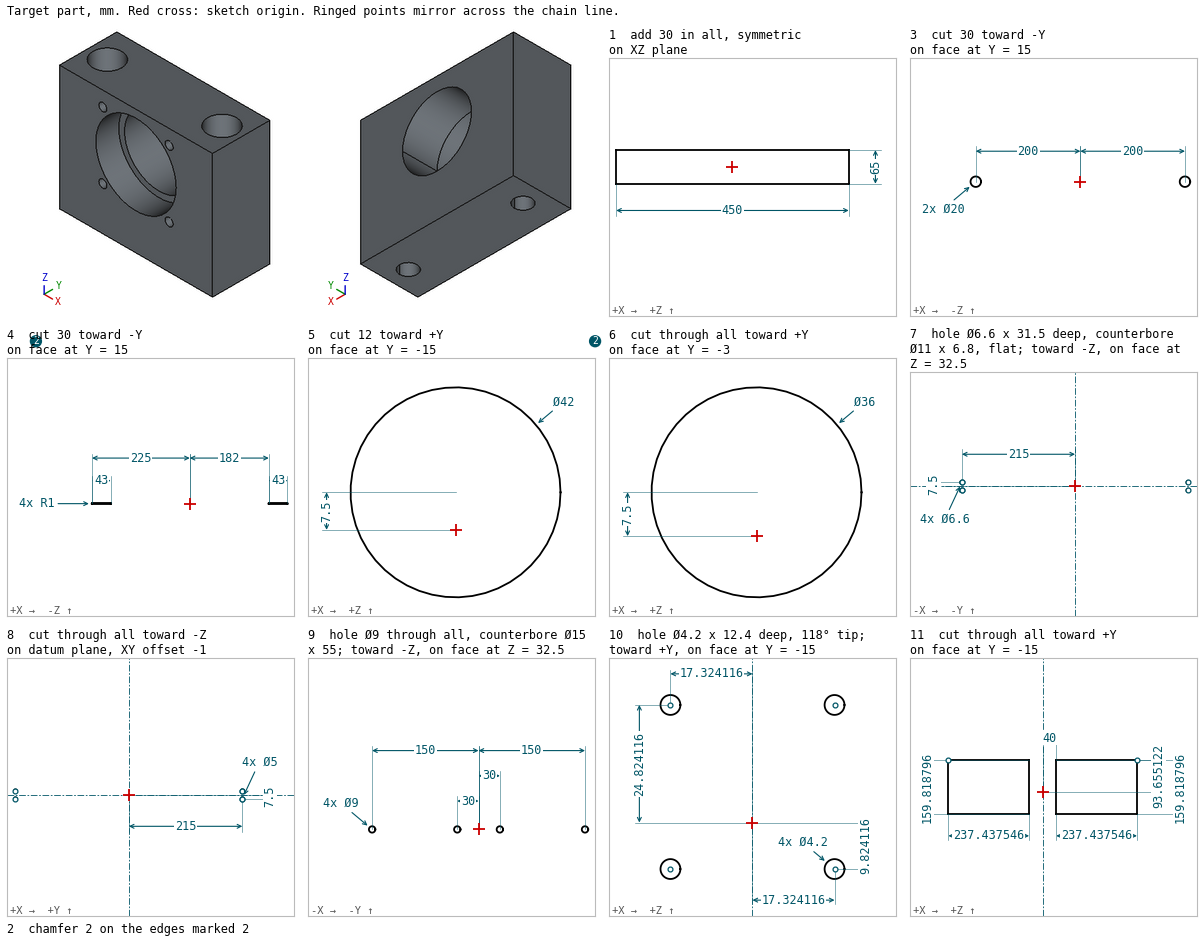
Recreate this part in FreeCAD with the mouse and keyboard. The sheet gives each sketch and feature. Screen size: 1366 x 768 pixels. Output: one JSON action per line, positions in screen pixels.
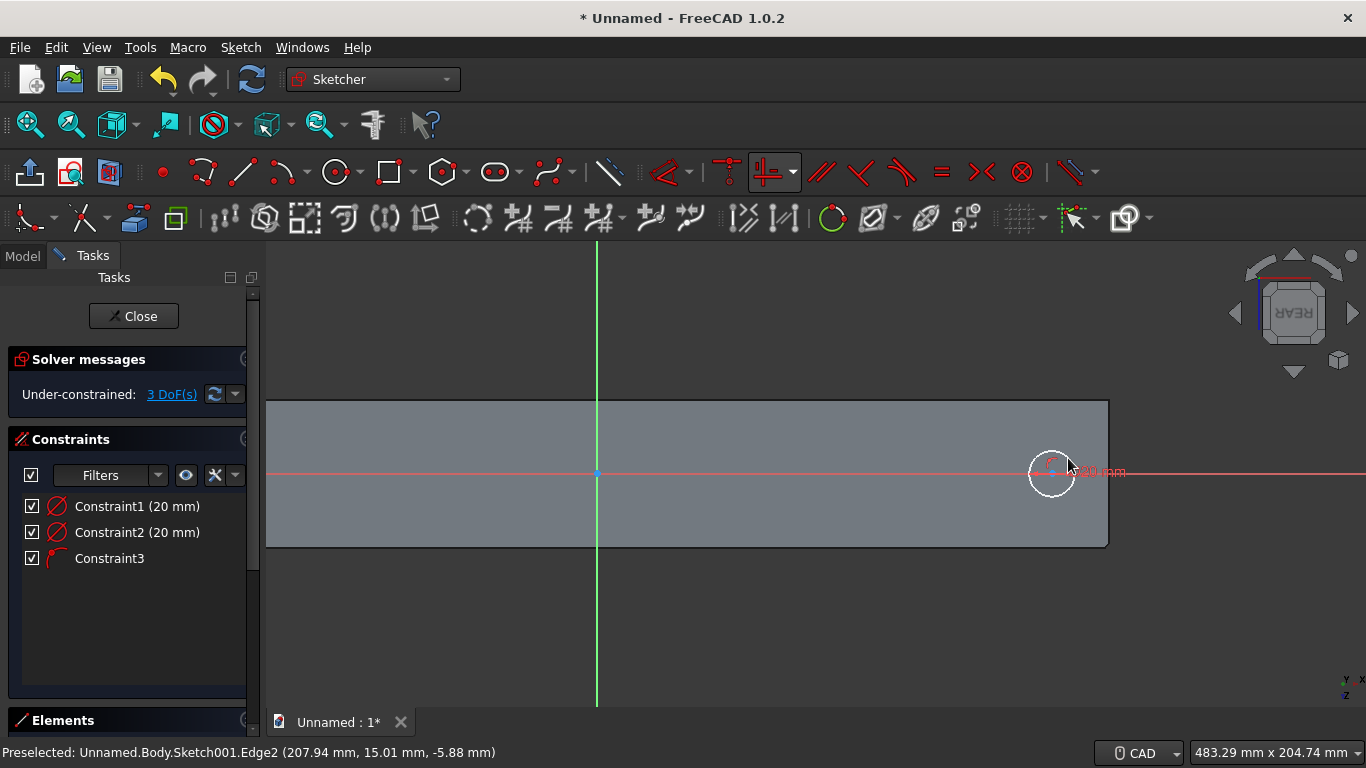
{"action": "scroll", "coordinate": [1053, 474], "scroll_direction": "down", "scroll_amount": 2}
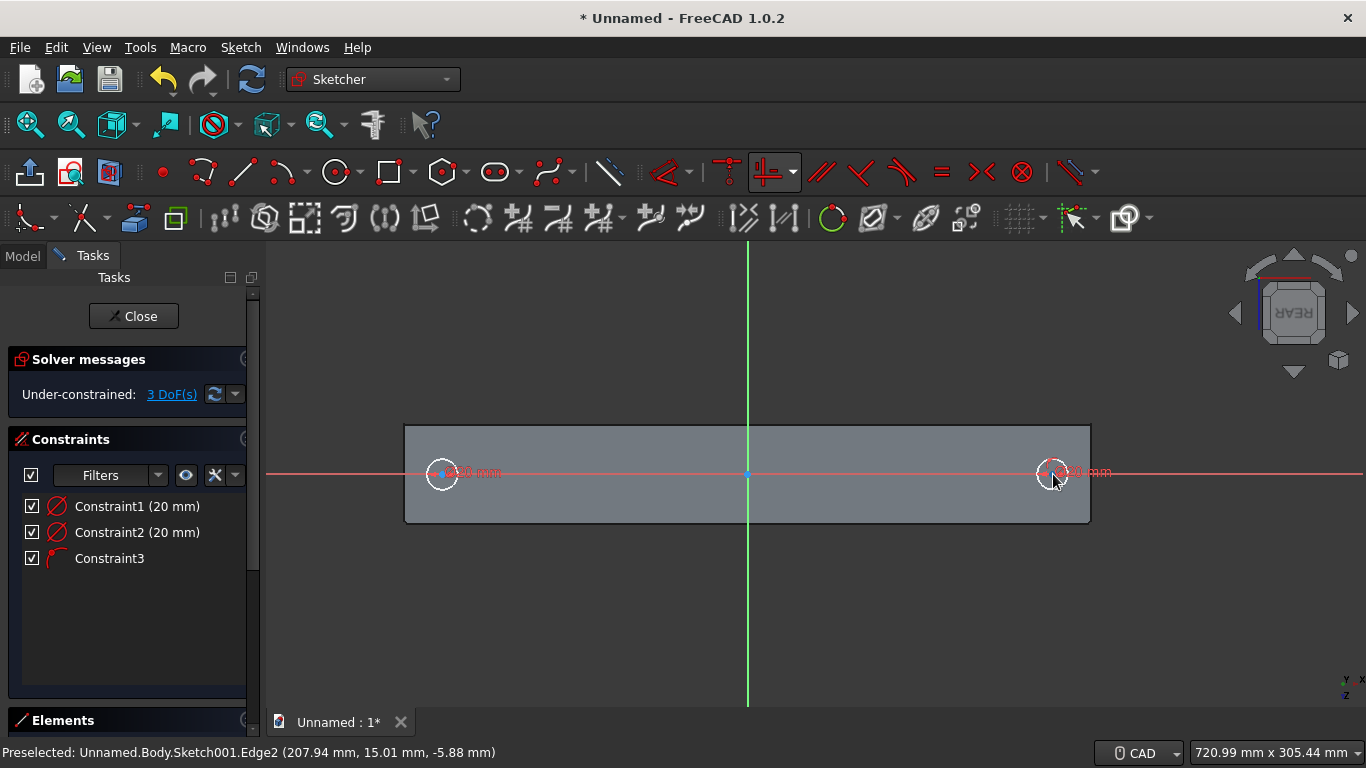
{"action": "left_click", "coordinate": [442, 474]}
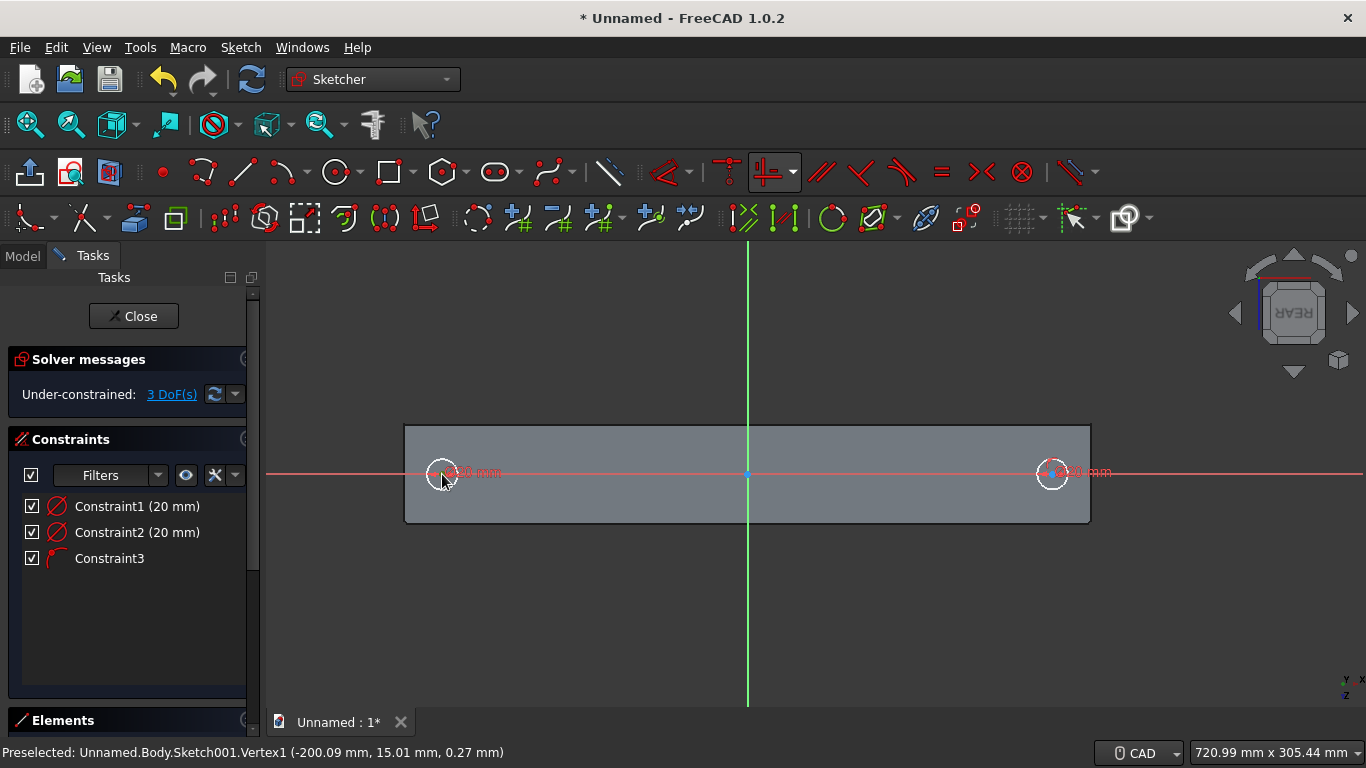
{"action": "left_click", "coordinate": [359, 474]}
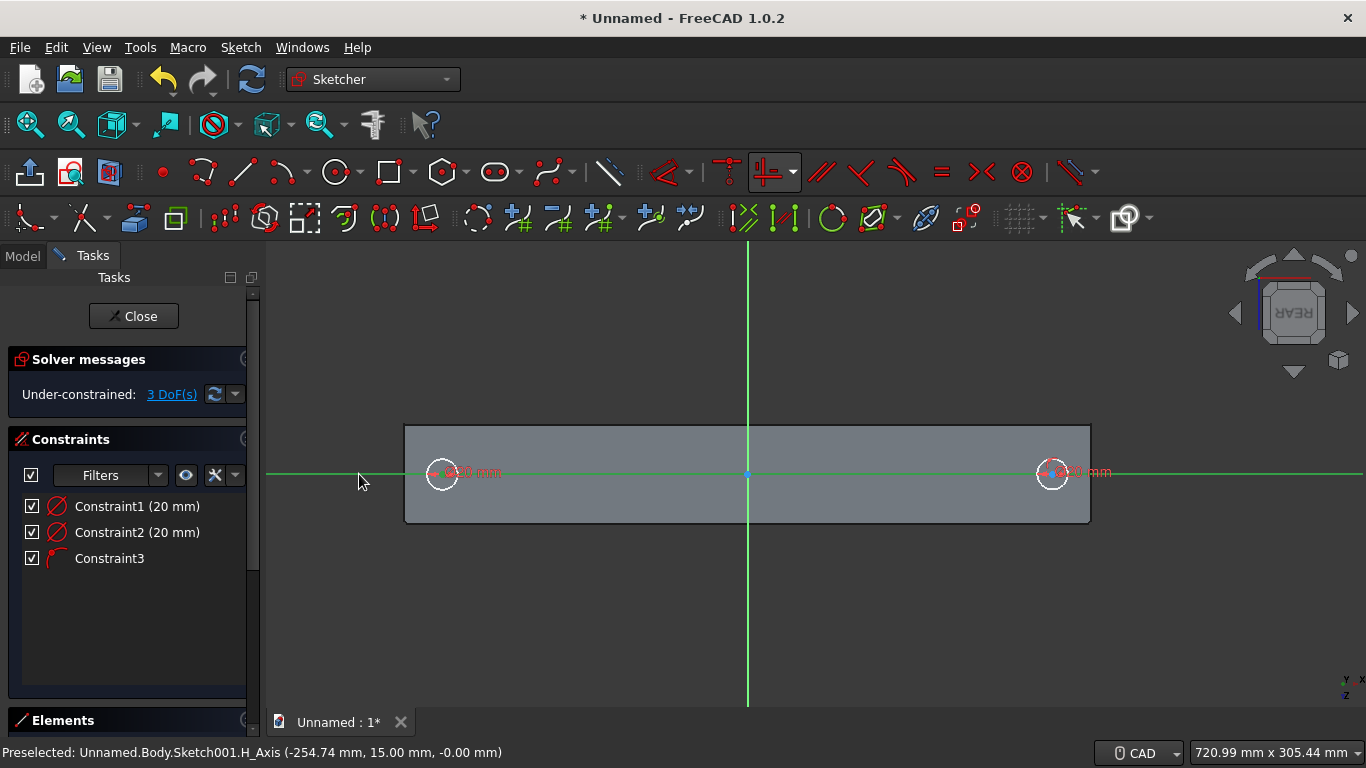
{"action": "key", "text": "c"}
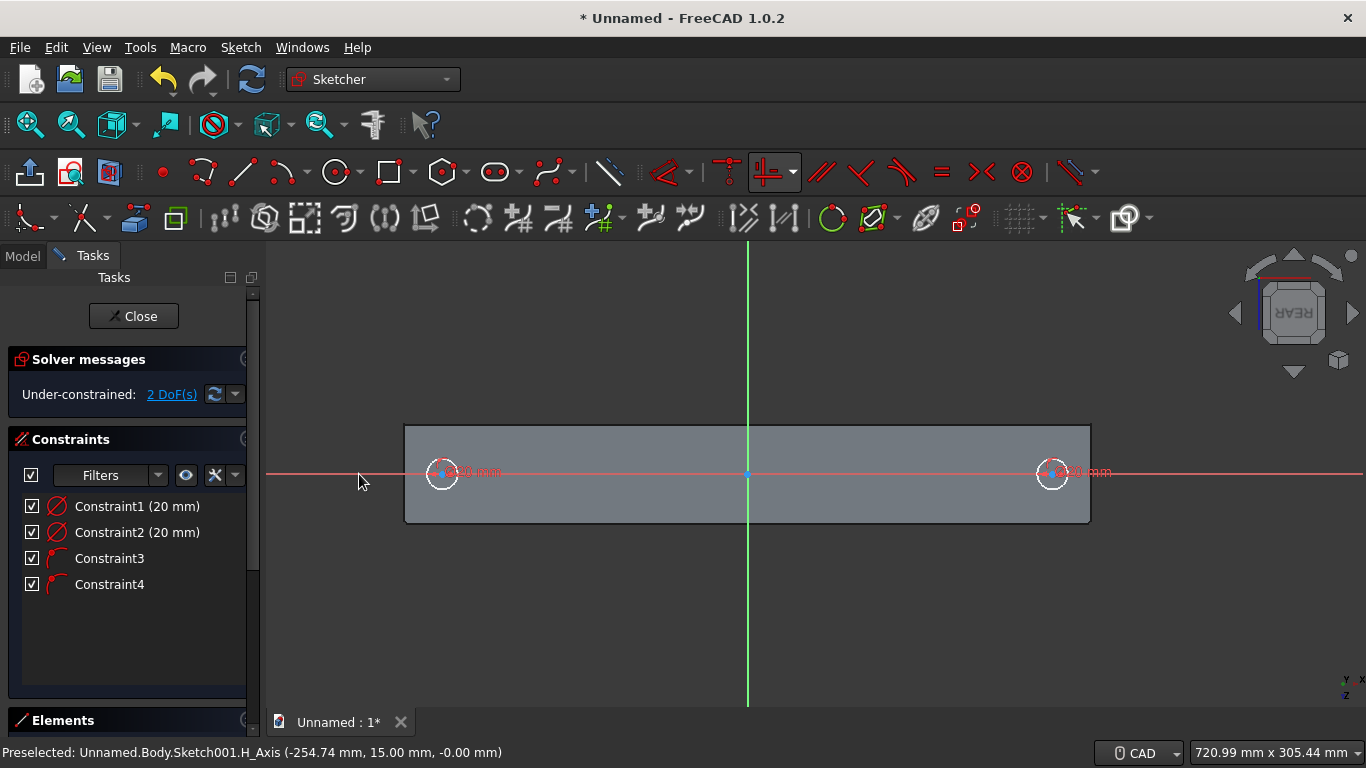
{"action": "key", "text": "d"}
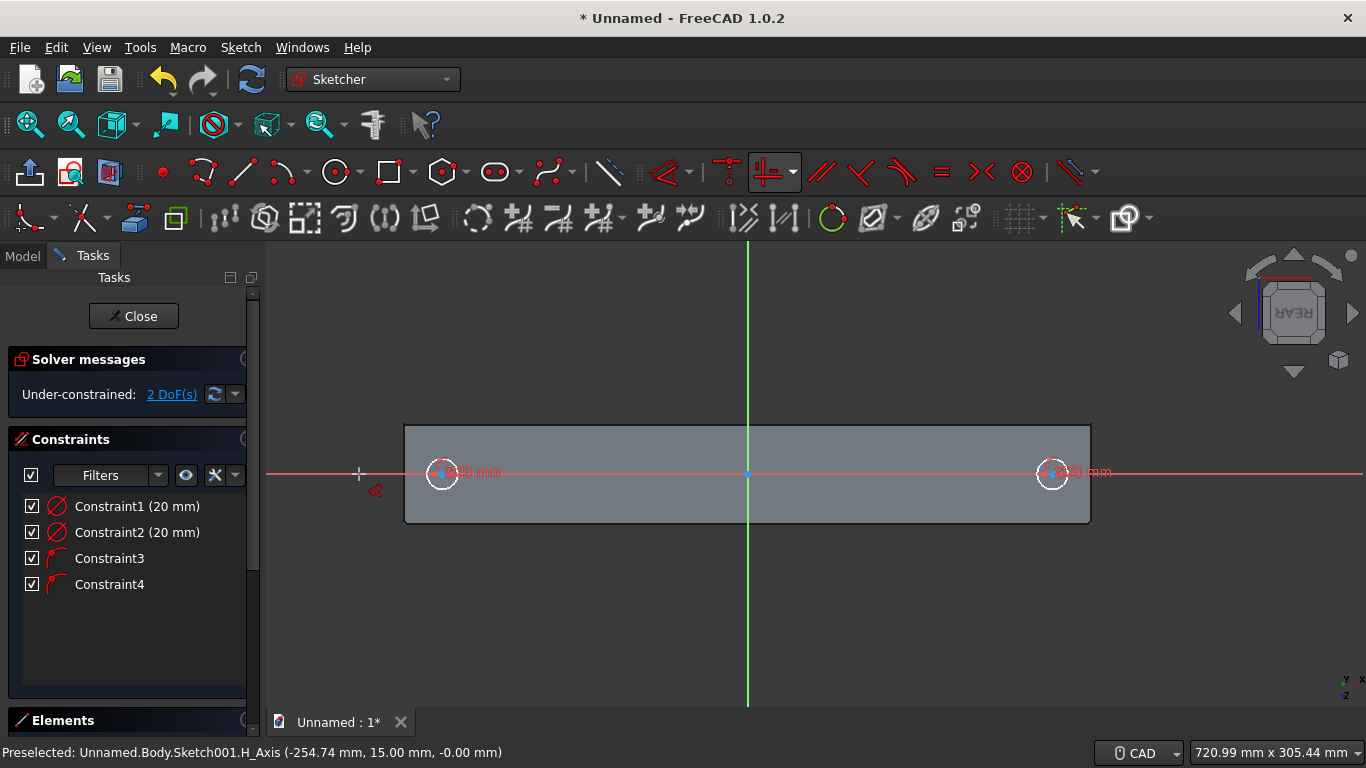
{"action": "left_click", "coordinate": [442, 474]}
{"action": "left_click", "coordinate": [595, 508]}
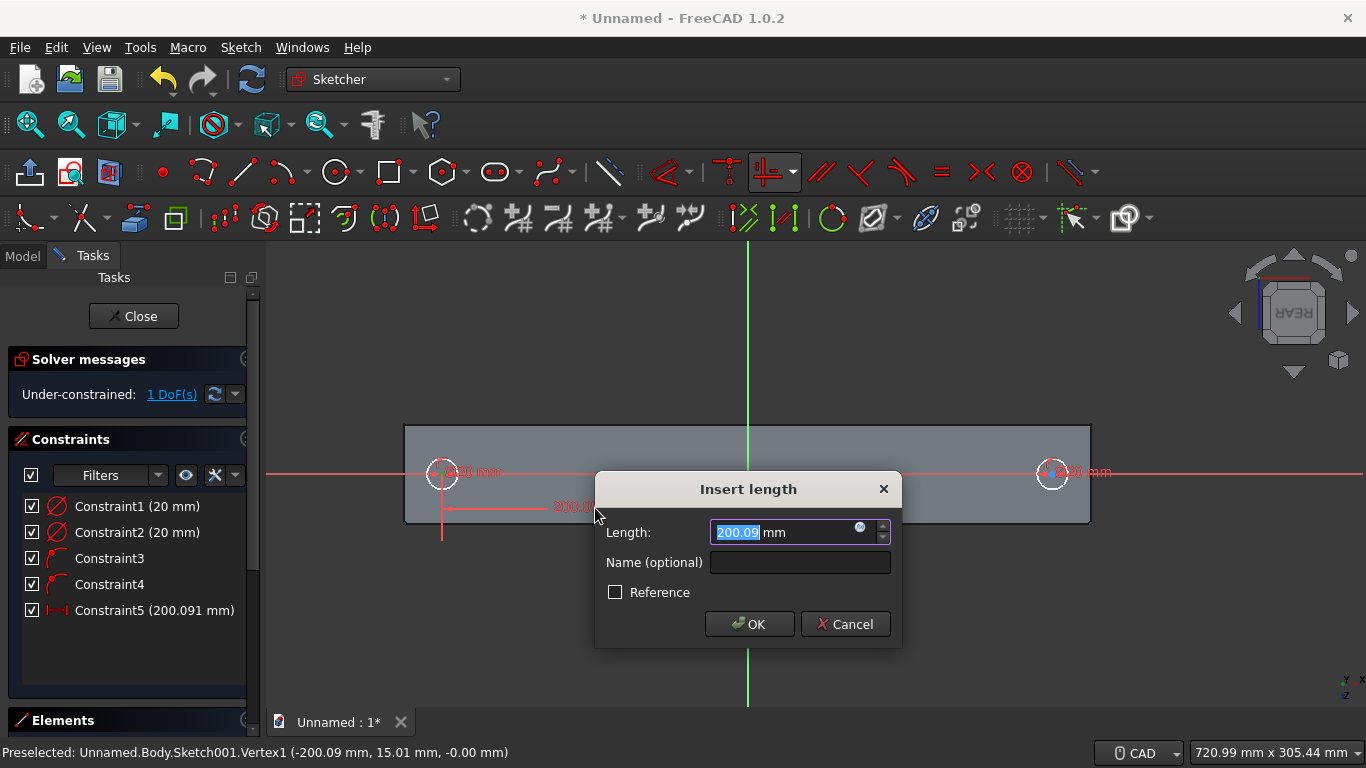
{"action": "type", "text": "200"}
{"action": "key", "text": "Return"}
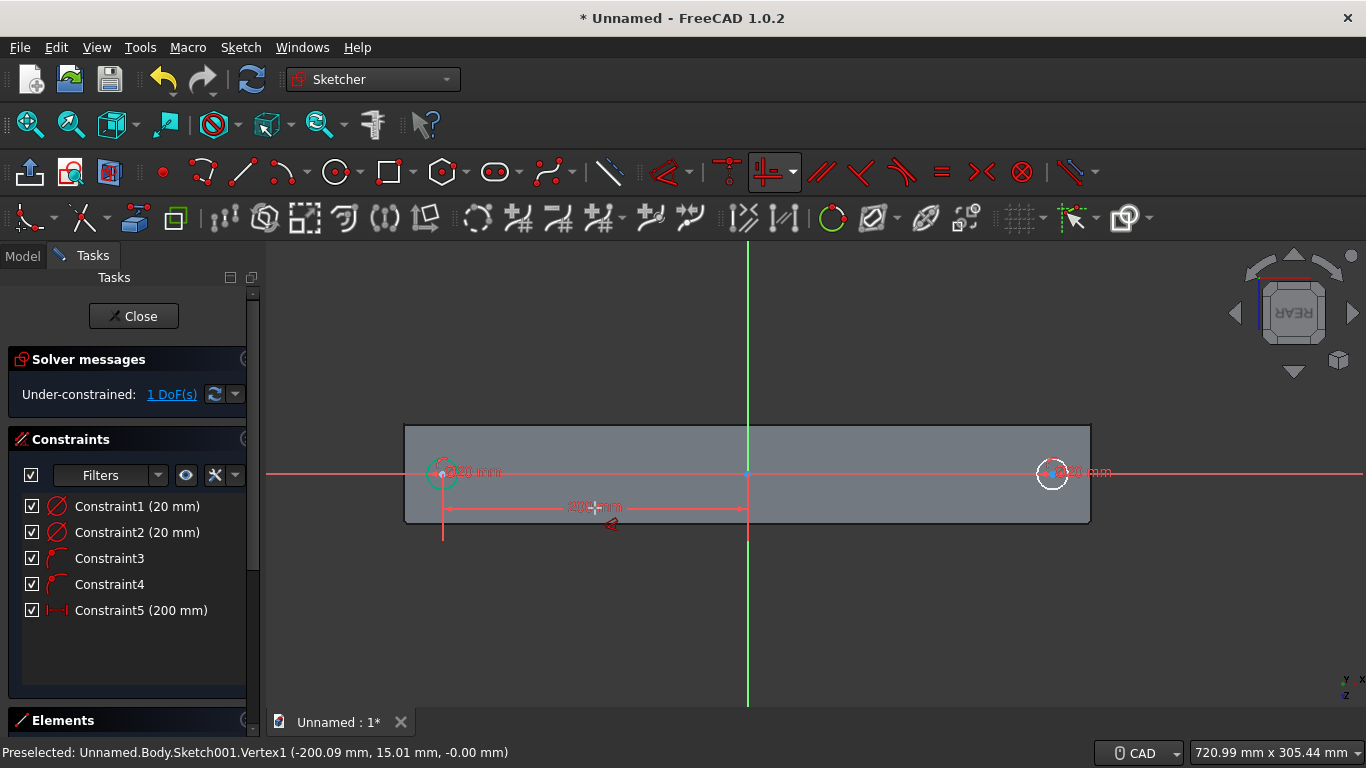
{"action": "left_click", "coordinate": [1053, 474]}
{"action": "left_click", "coordinate": [900, 508]}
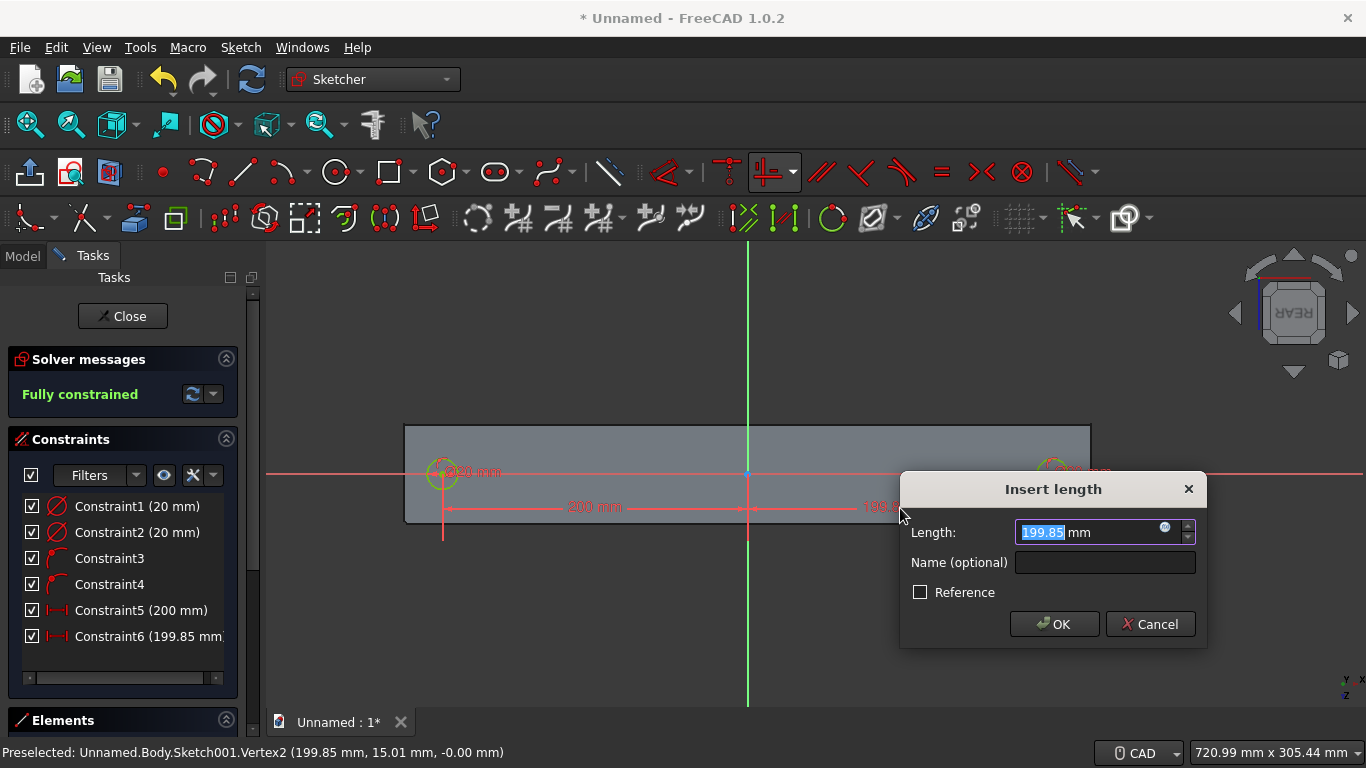
{"action": "type", "text": "200"}
{"action": "key", "text": "Return"}
{"action": "key", "text": "Escape"}